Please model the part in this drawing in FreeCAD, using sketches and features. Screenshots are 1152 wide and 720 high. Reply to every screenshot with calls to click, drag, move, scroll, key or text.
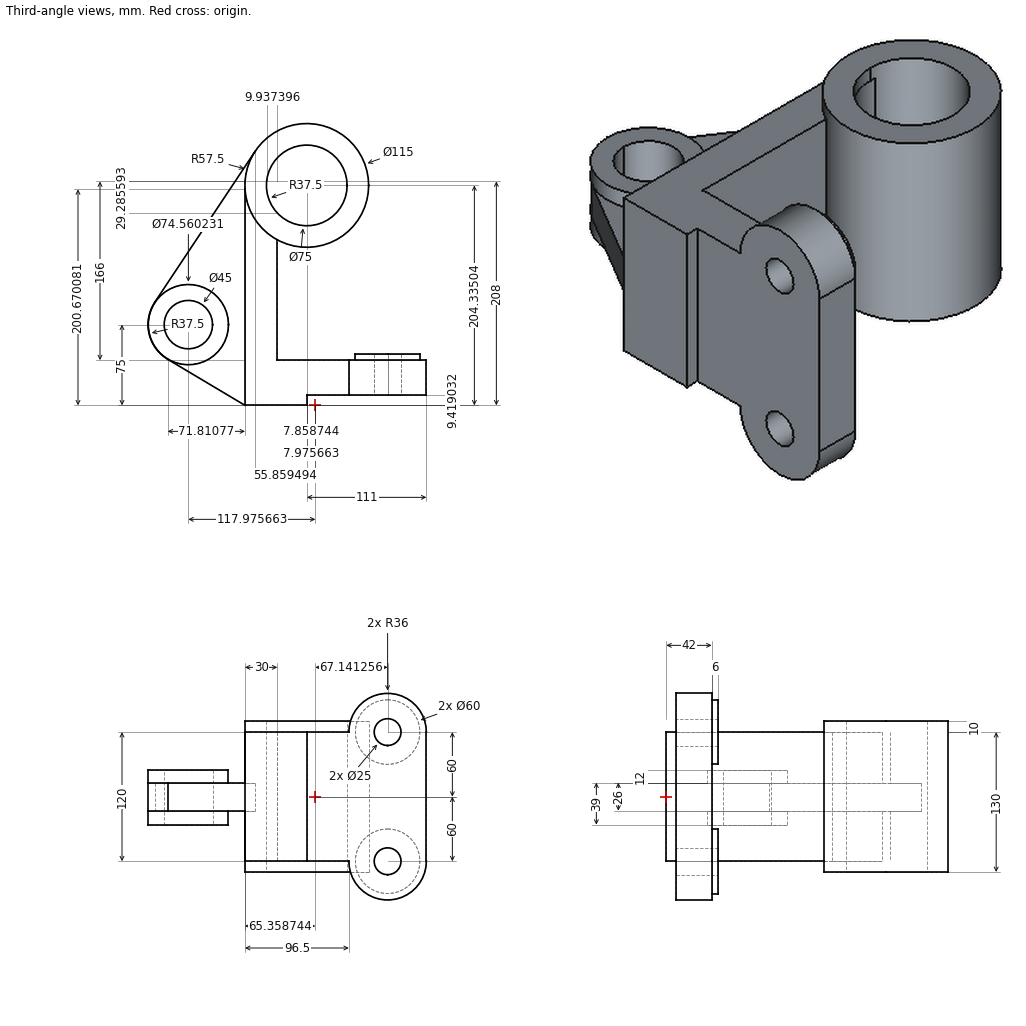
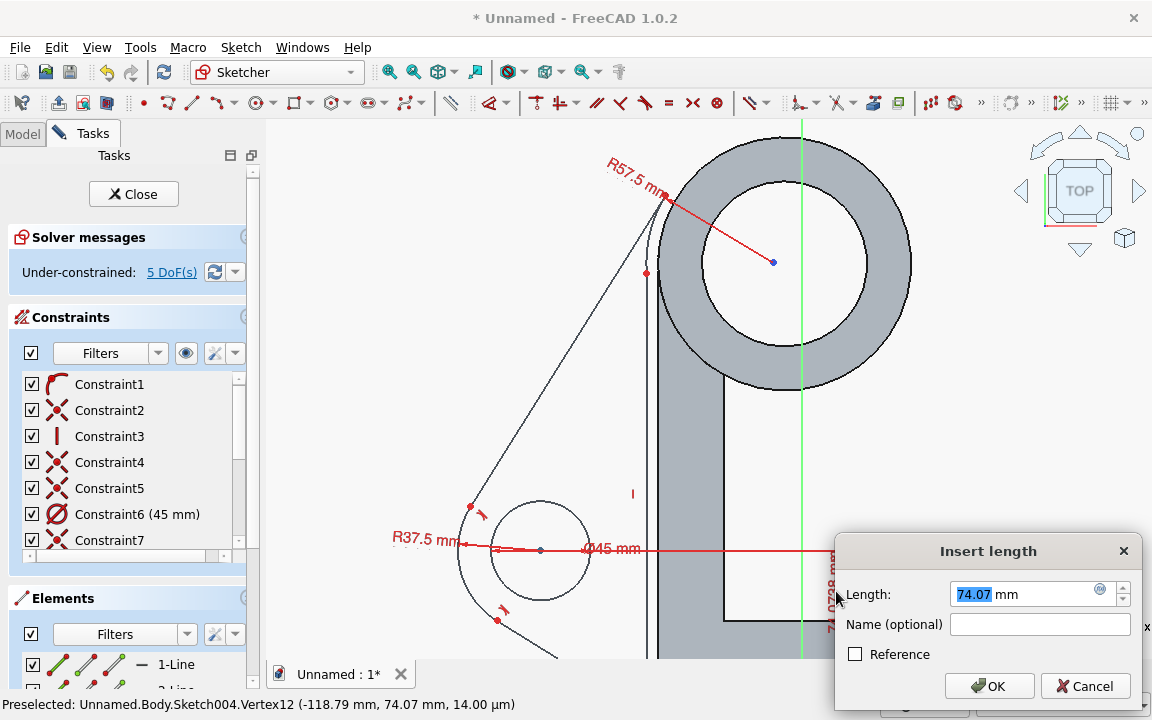
text(75)
key(Return)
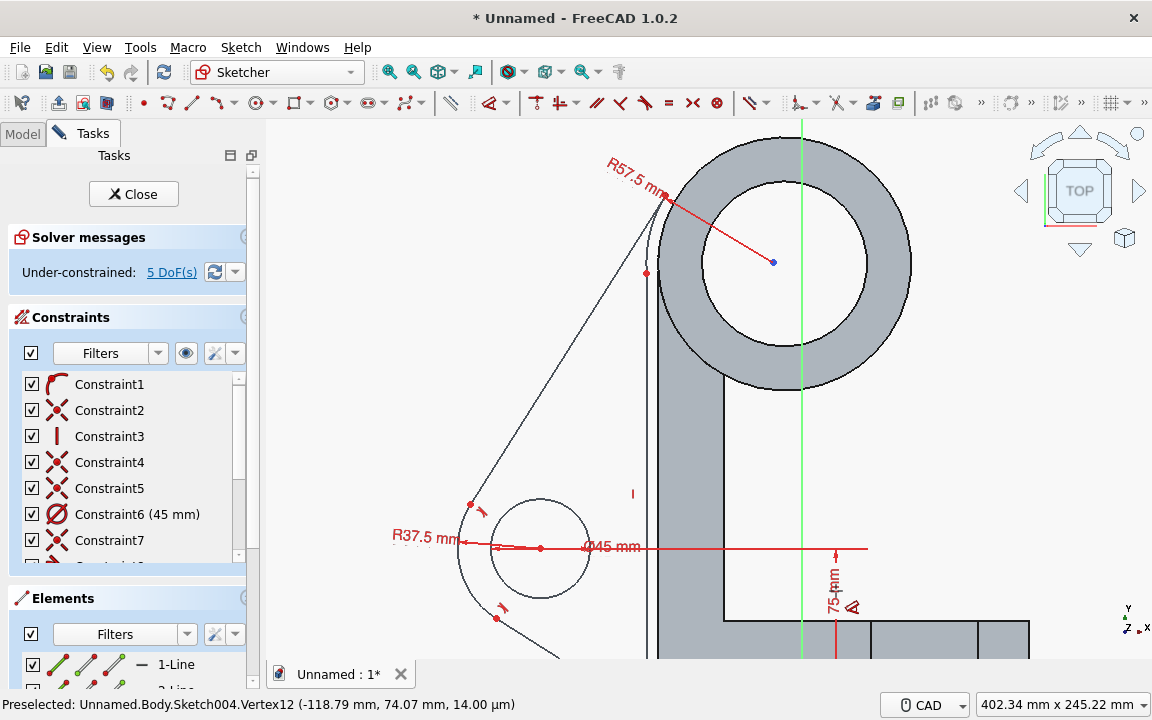
scroll(658, 257, down, 2)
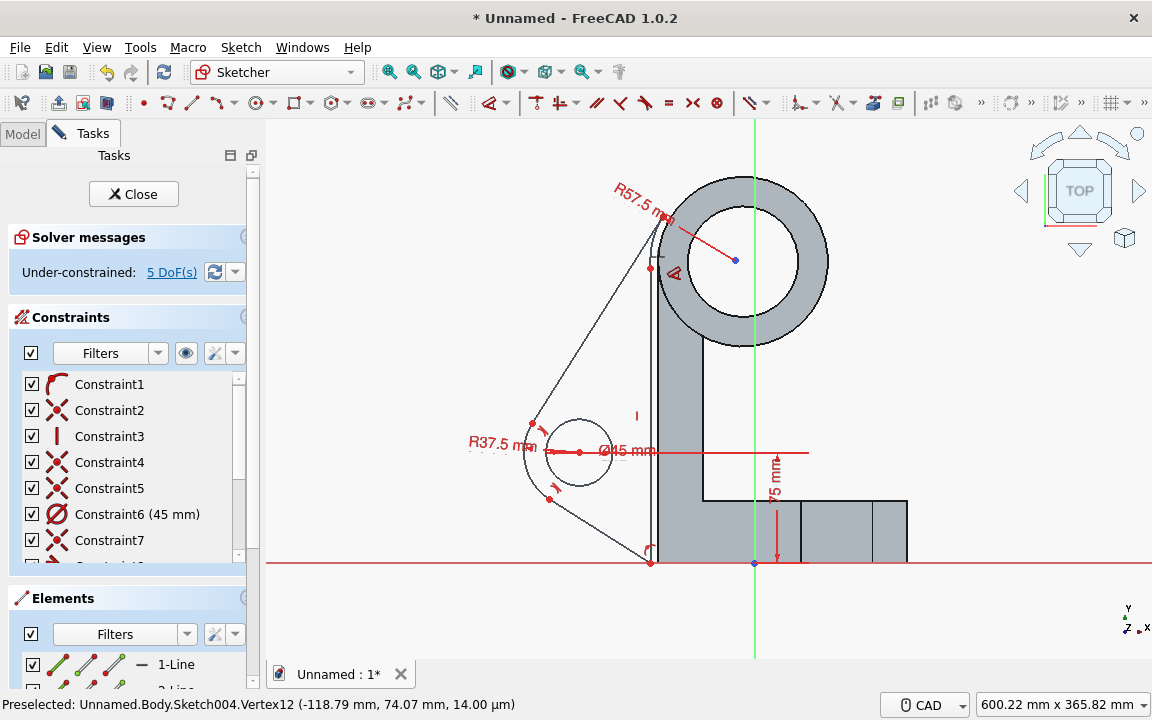
click(580, 519)
click(600, 597)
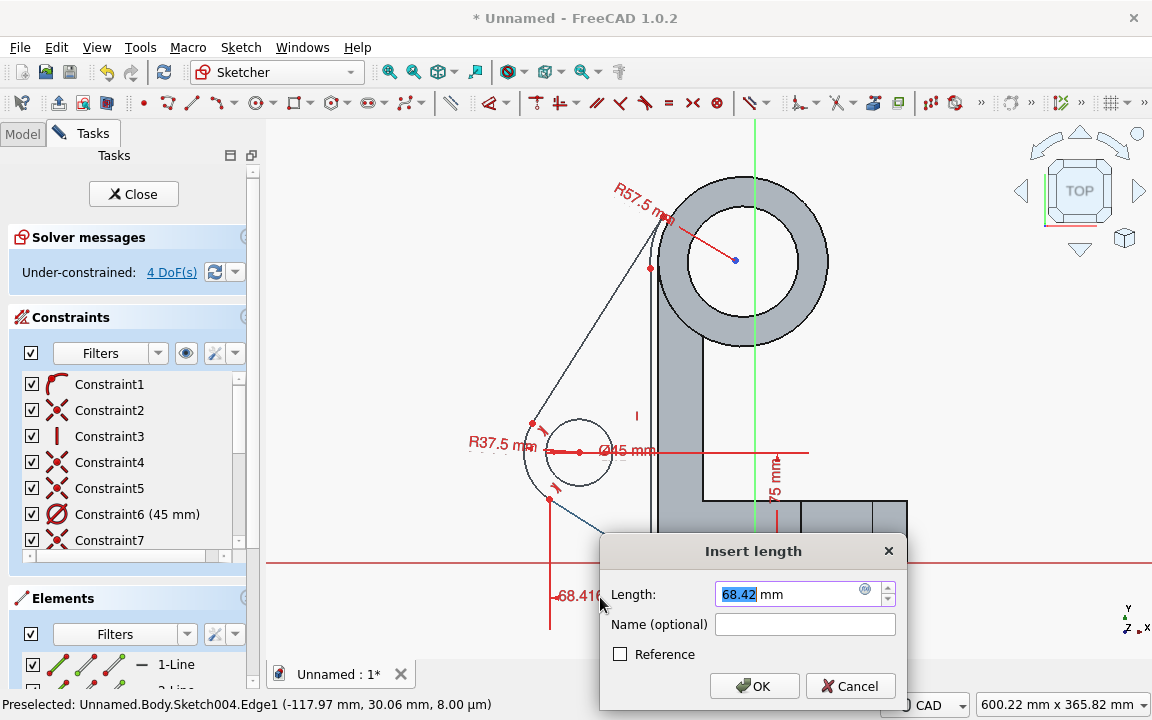
text(71.81077)
key(Return)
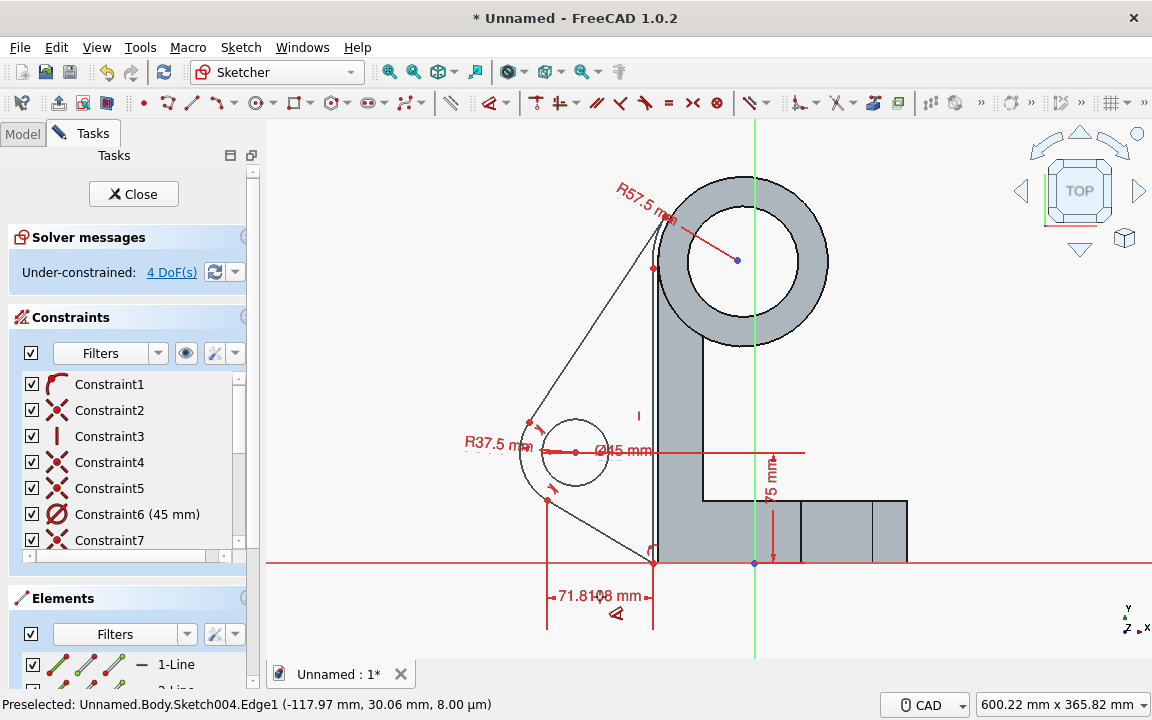
scroll(738, 261, up, 7)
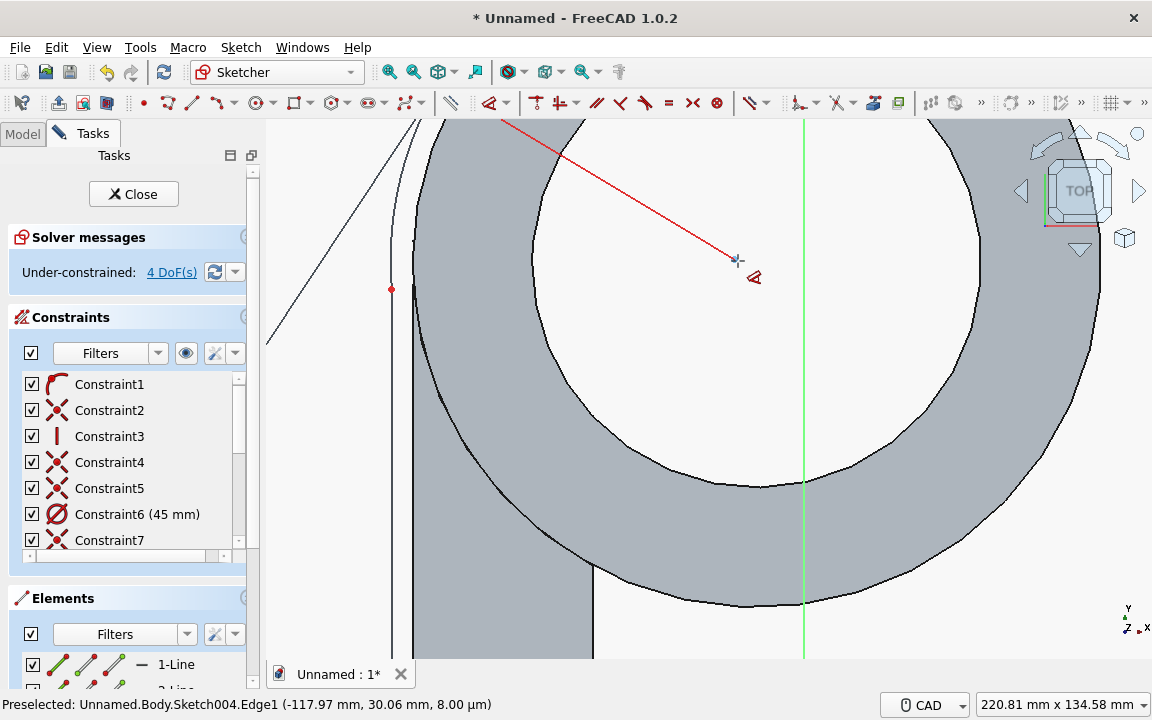
click(735, 260)
click(770, 226)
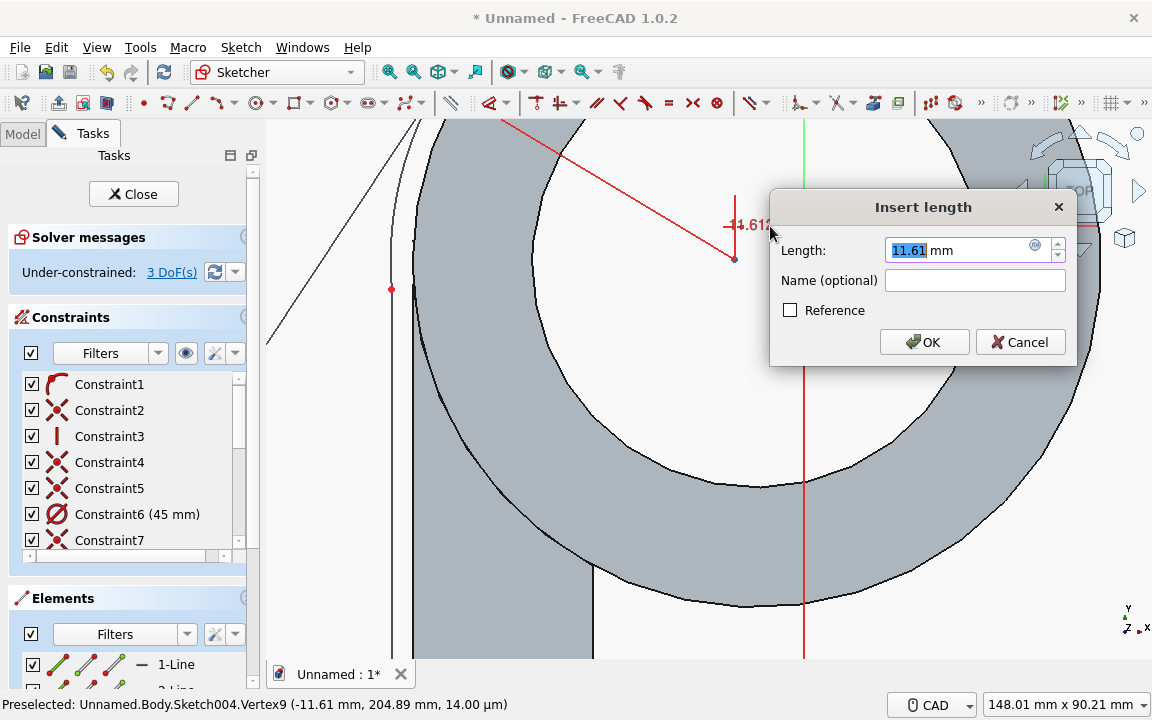
text(7.975663)
key(Return)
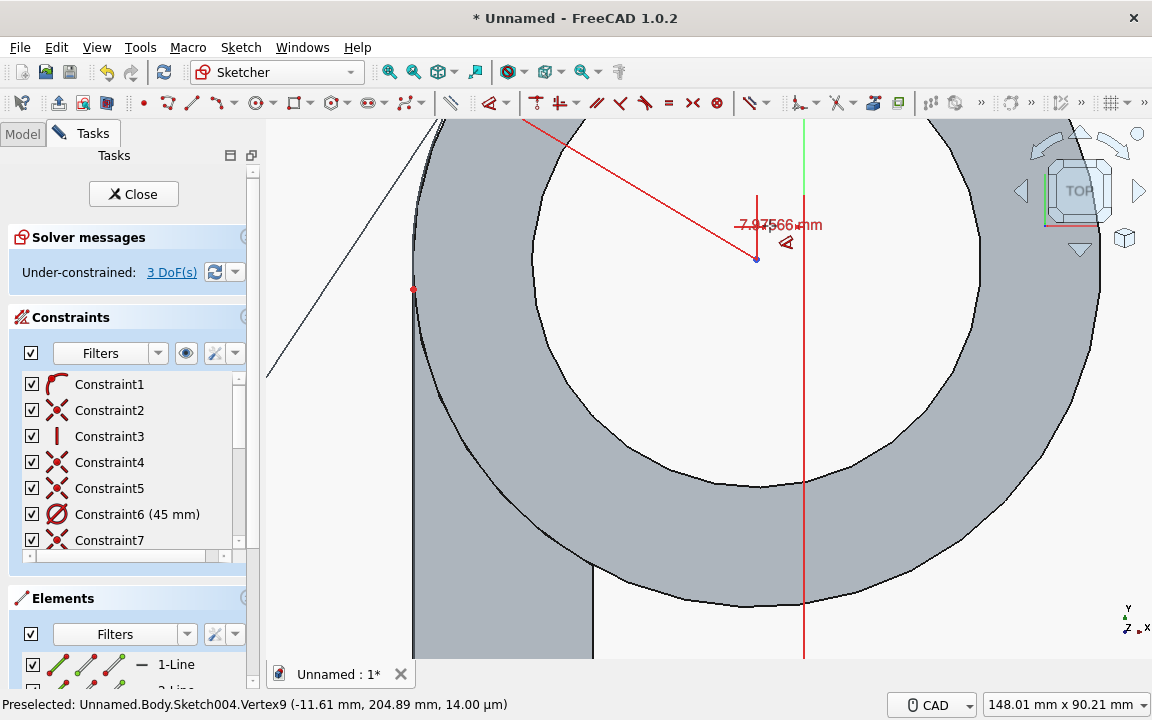
scroll(738, 261, down, 7)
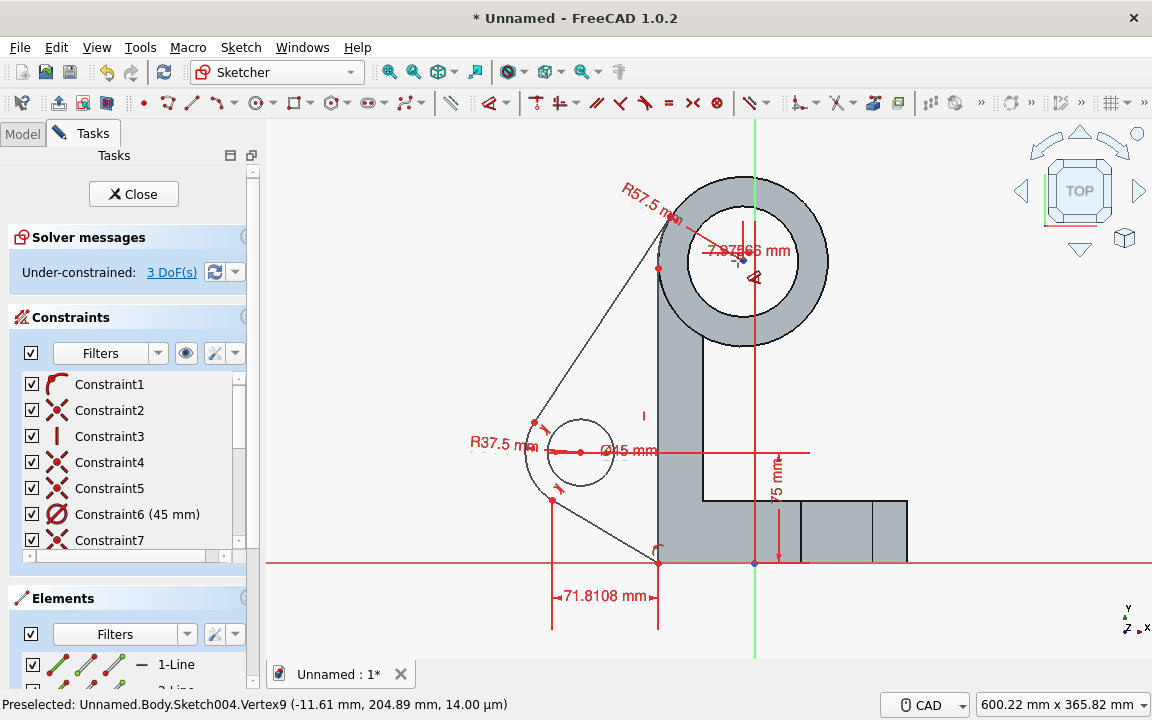
click(658, 327)
click(692, 416)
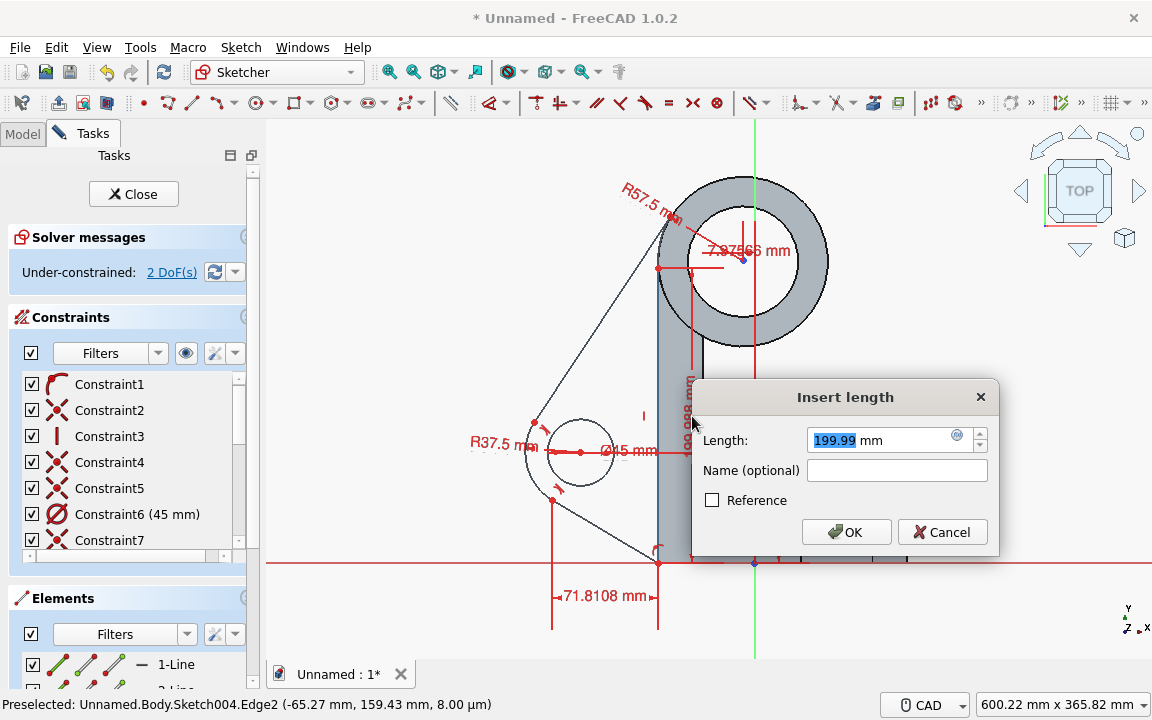
text(200.670081)
key(Return)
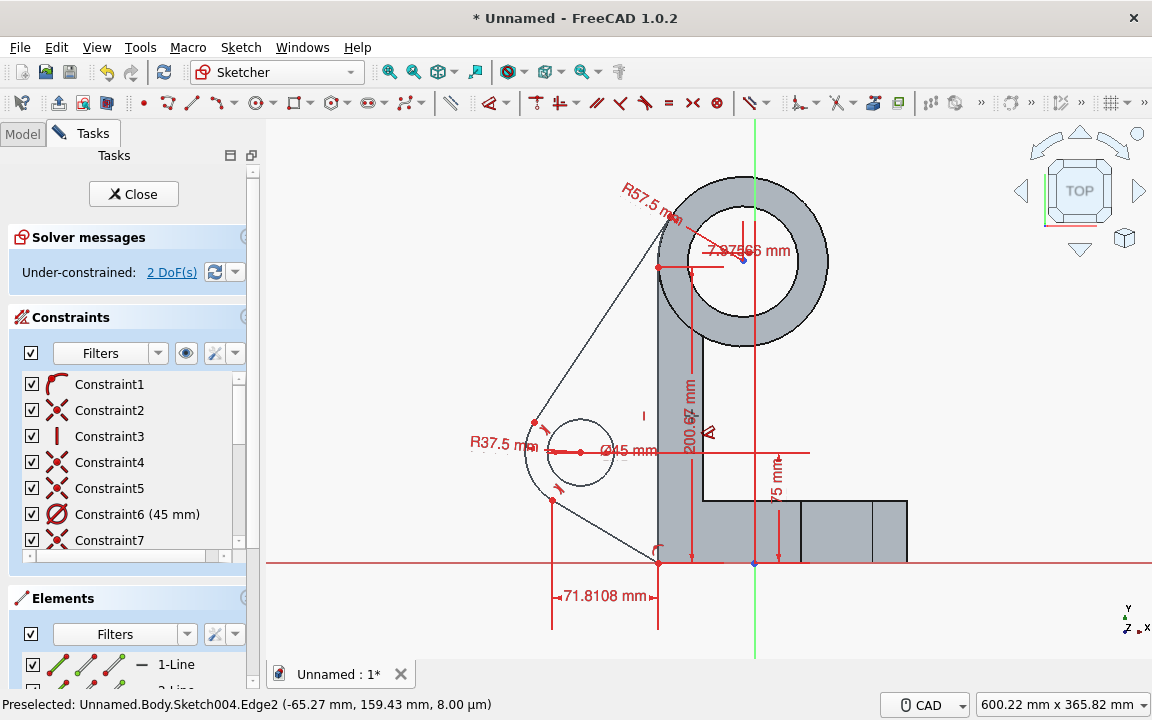
click(671, 216)
click(713, 597)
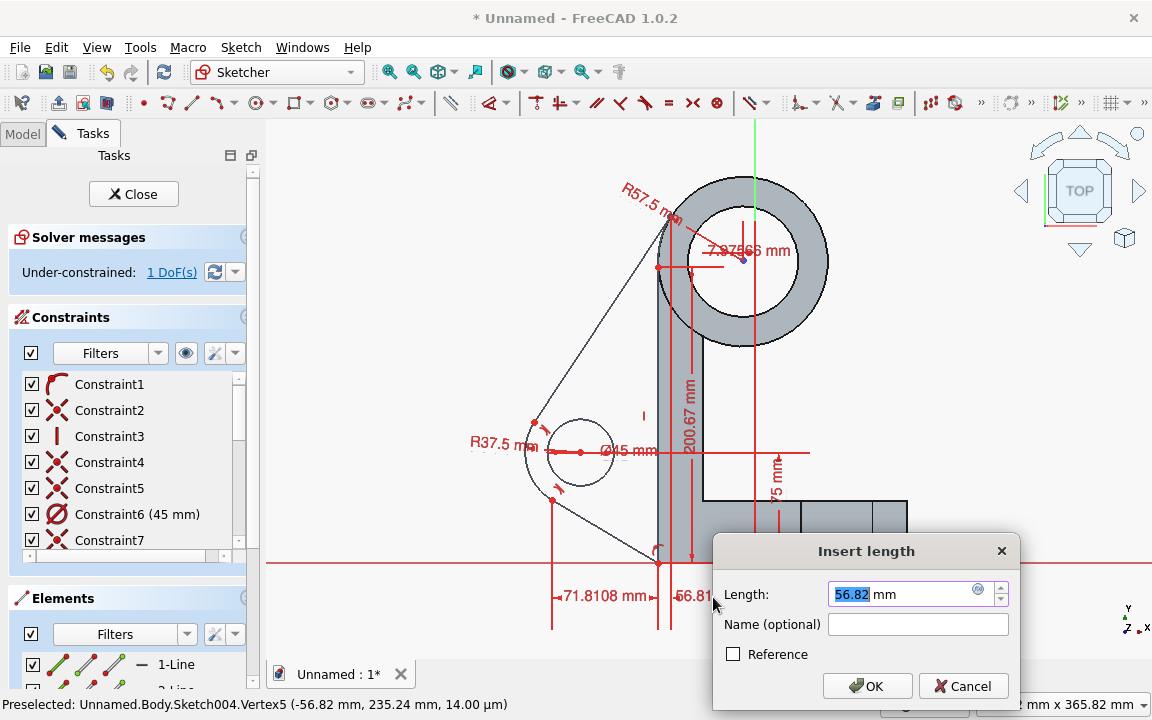
text(55.859494)
key(Return)